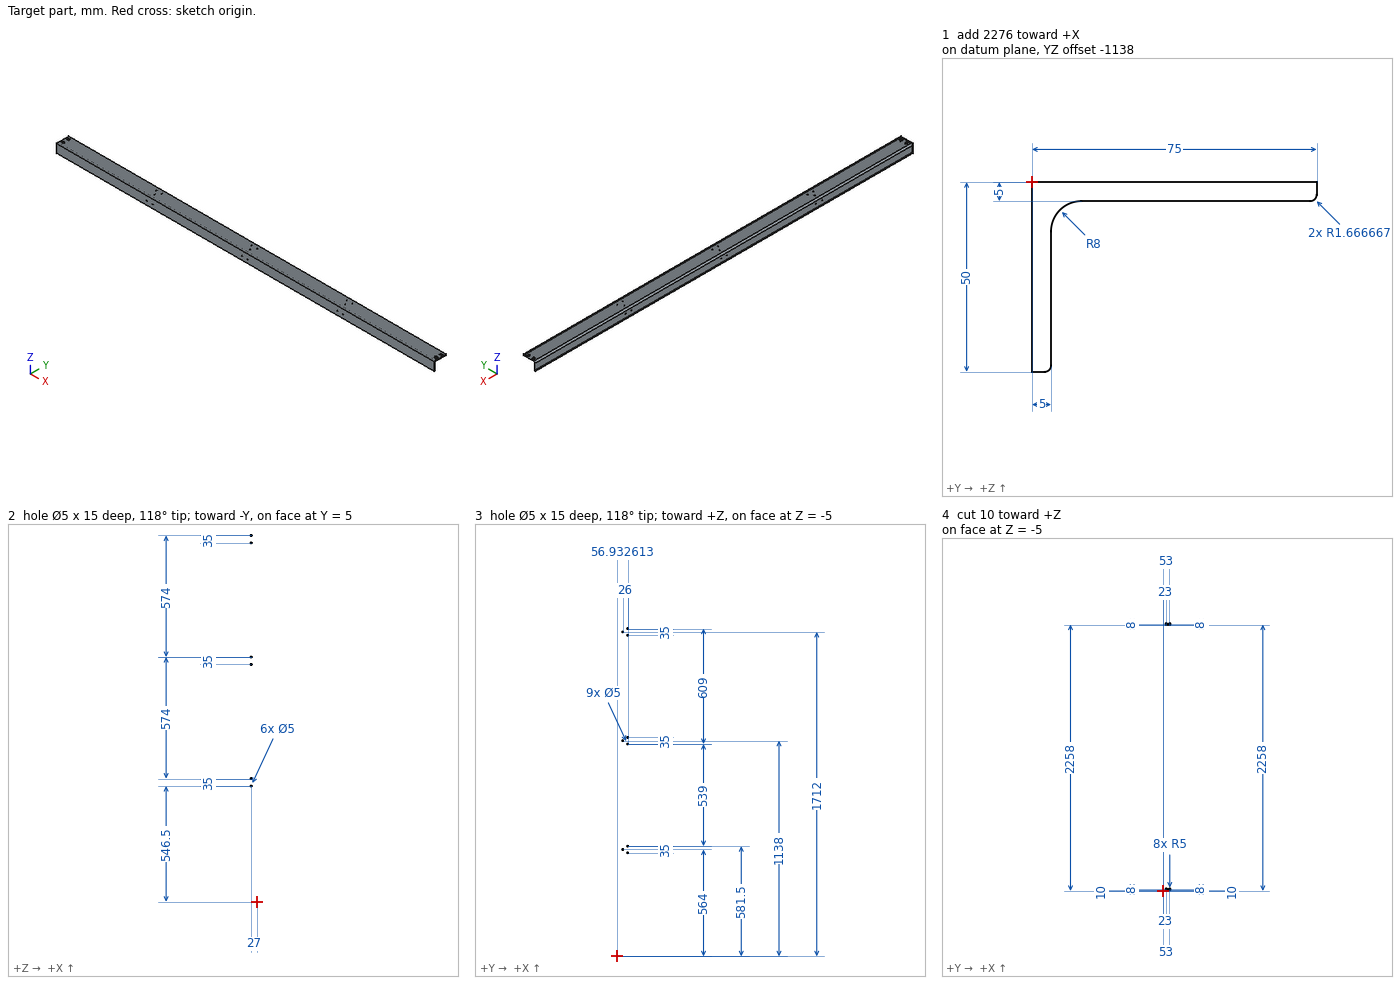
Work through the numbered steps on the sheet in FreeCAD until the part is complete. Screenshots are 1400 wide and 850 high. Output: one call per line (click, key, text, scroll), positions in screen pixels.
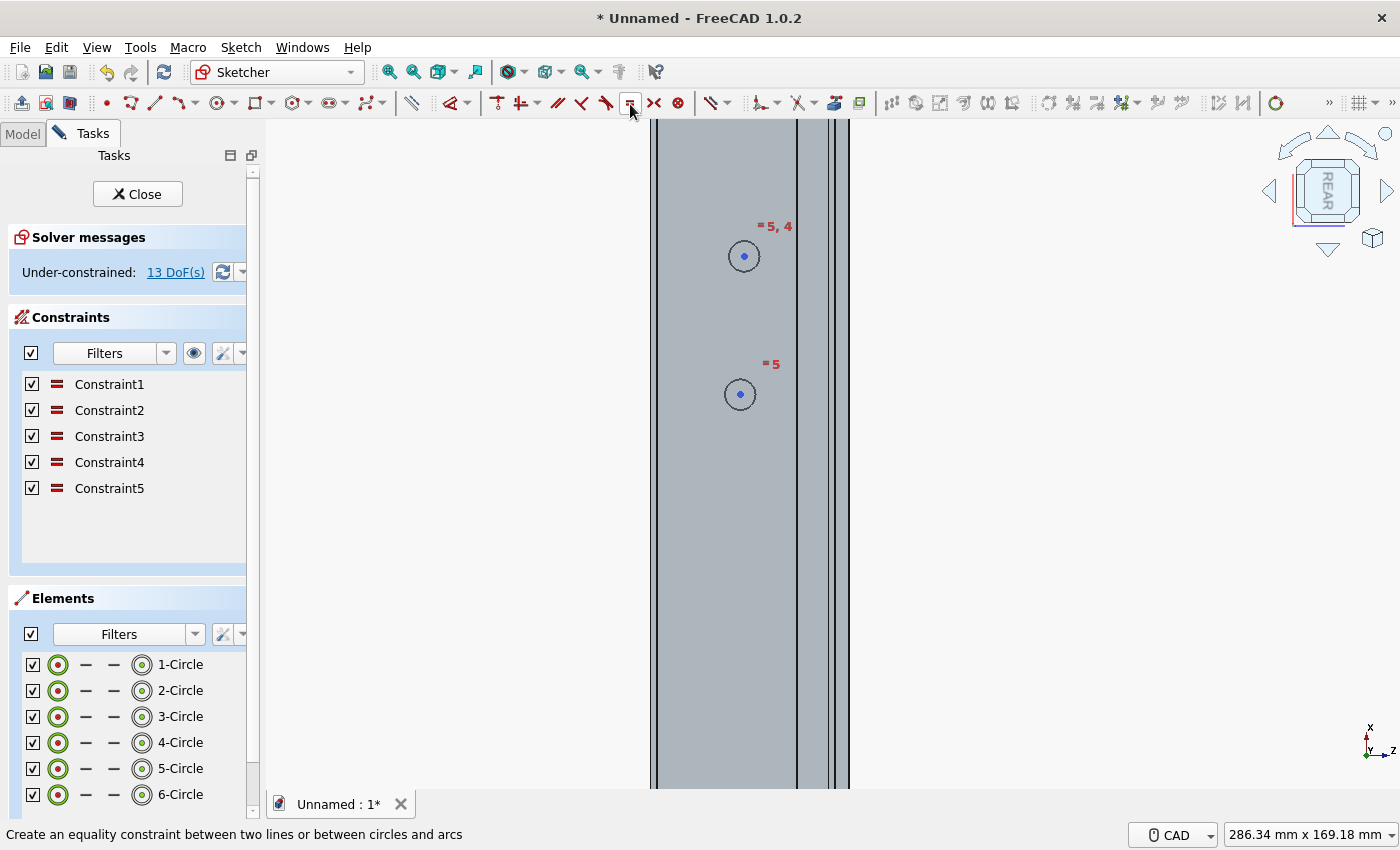
scroll(763, 246, down, 14)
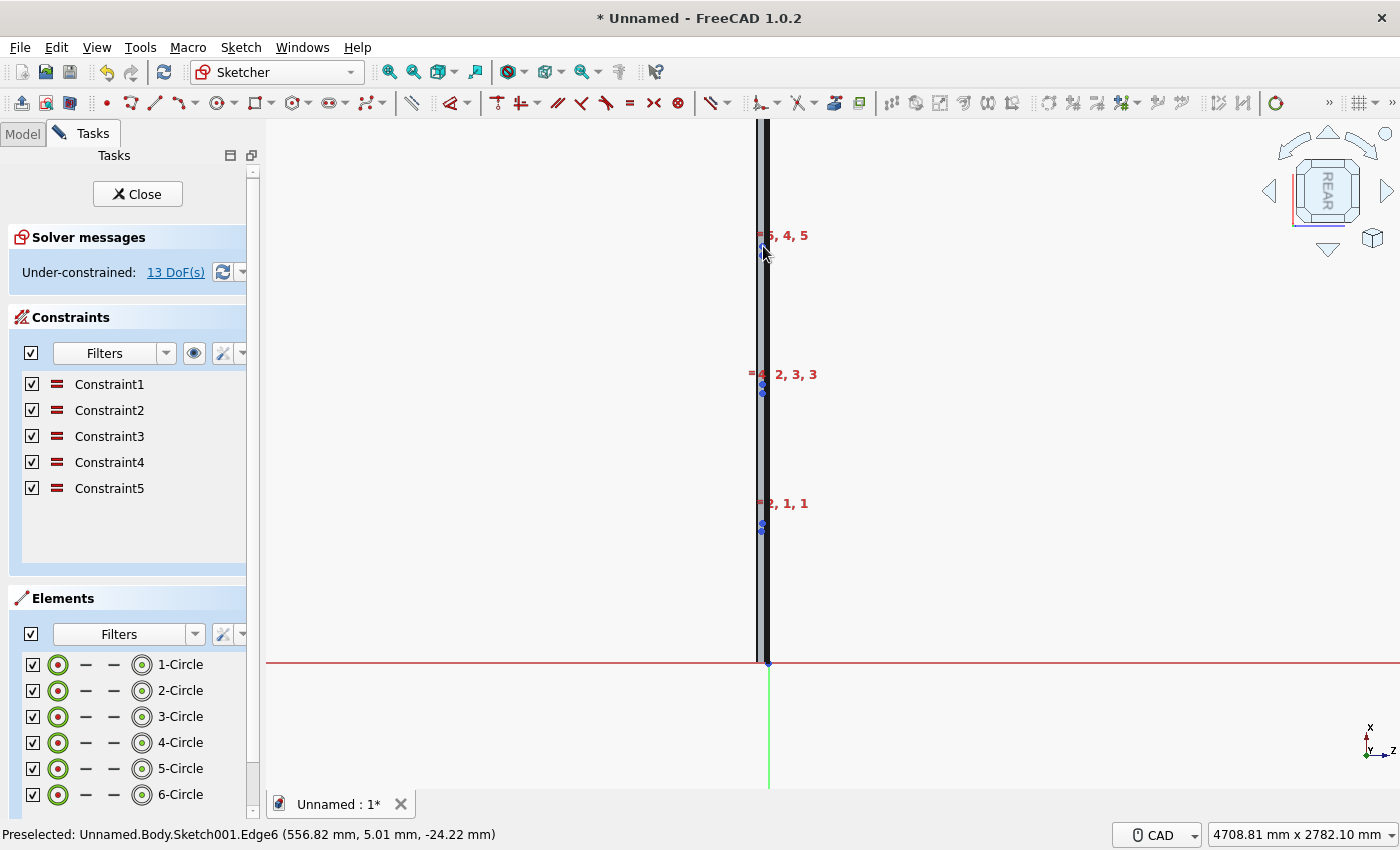
scroll(762, 532, up, 2)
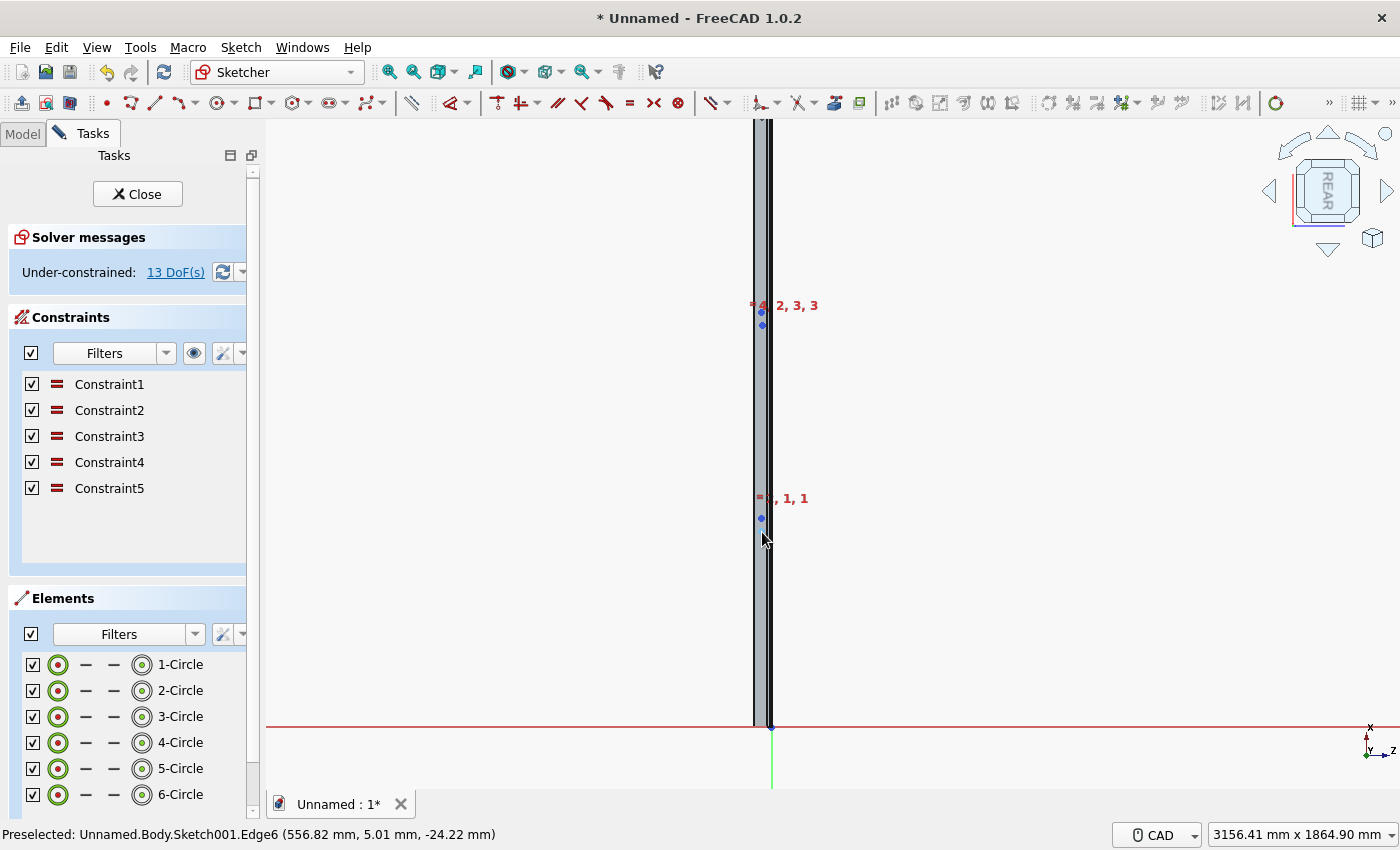
click(762, 531)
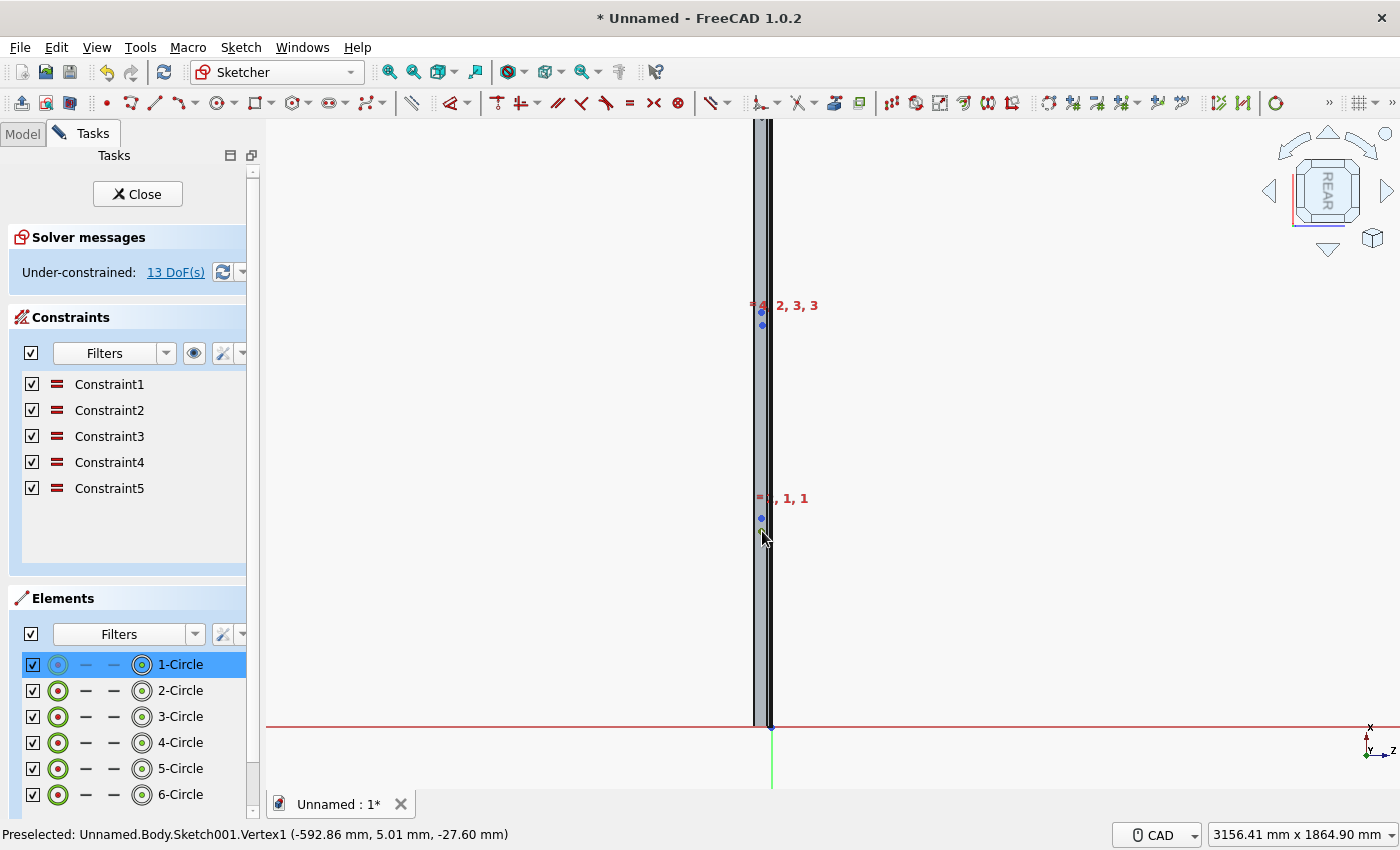
click(762, 519)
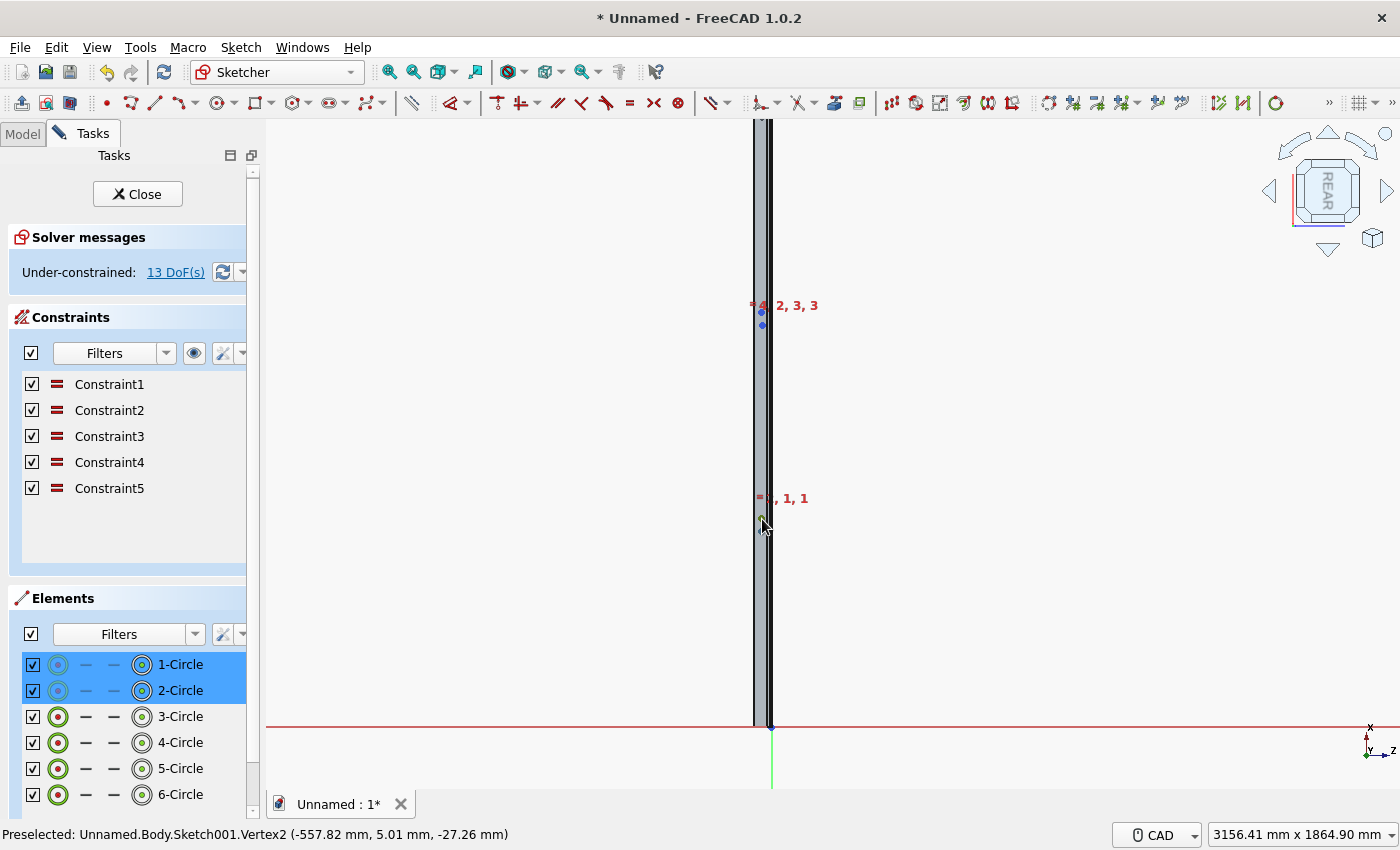
click(540, 104)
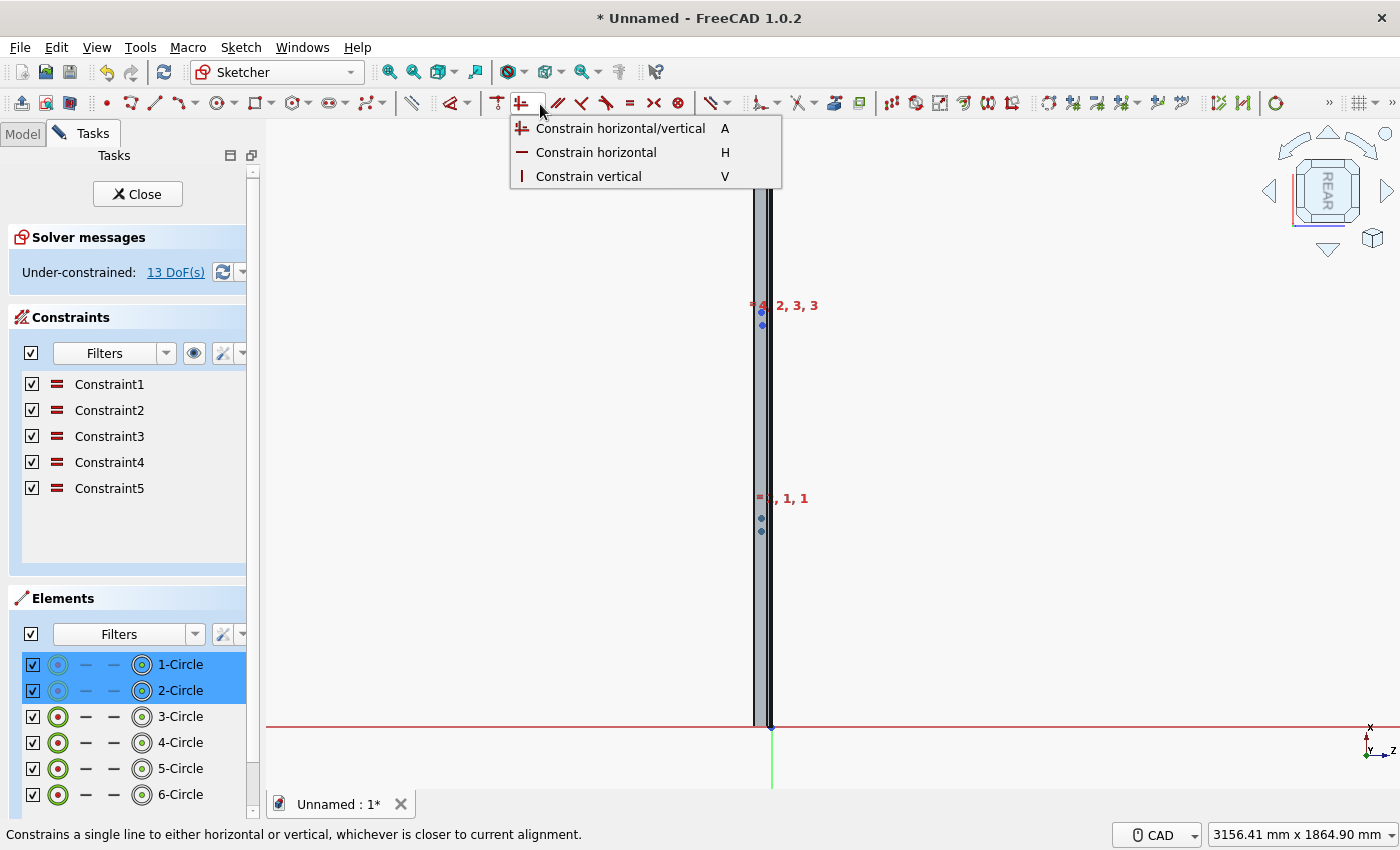
click(646, 176)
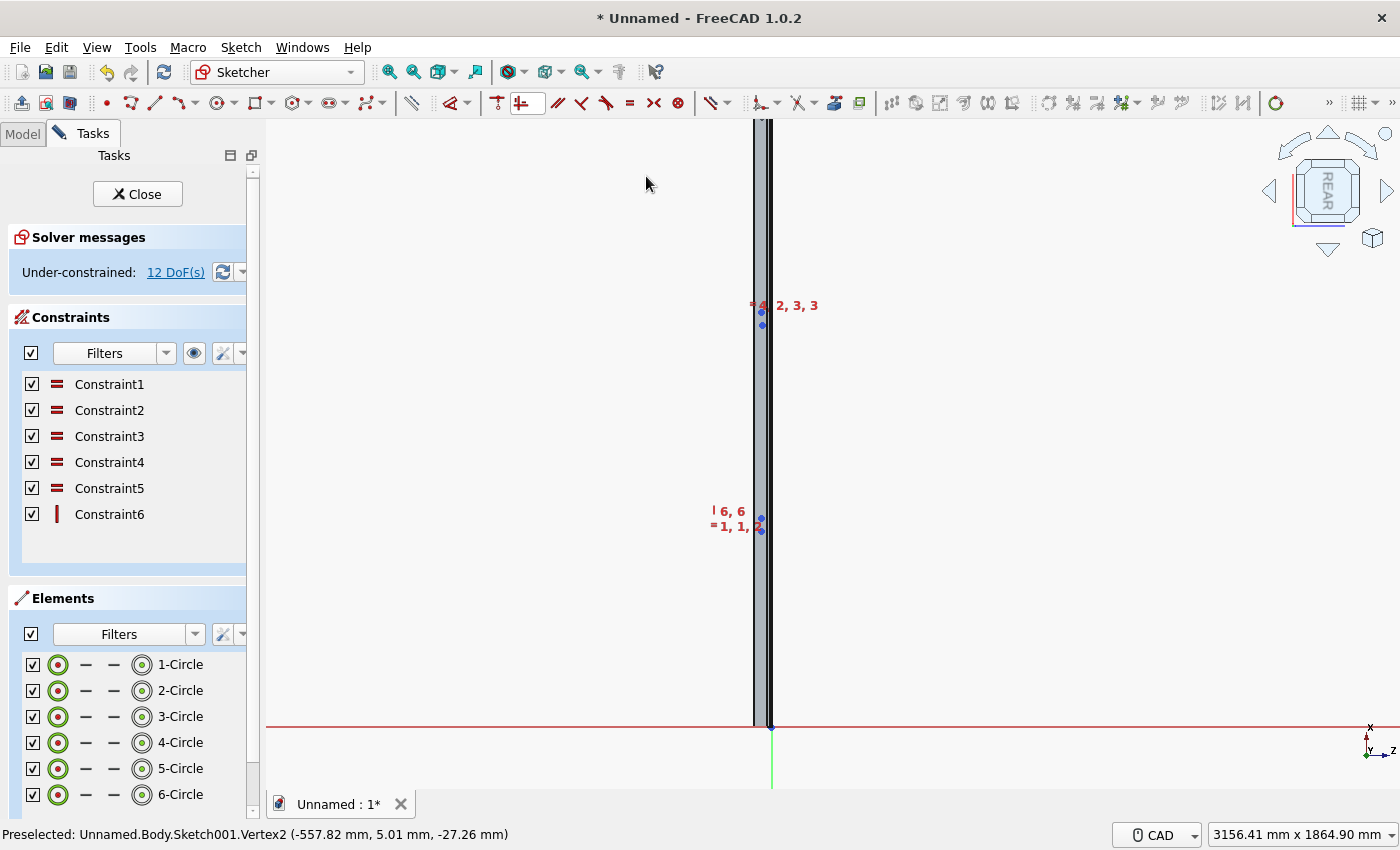
click(762, 519)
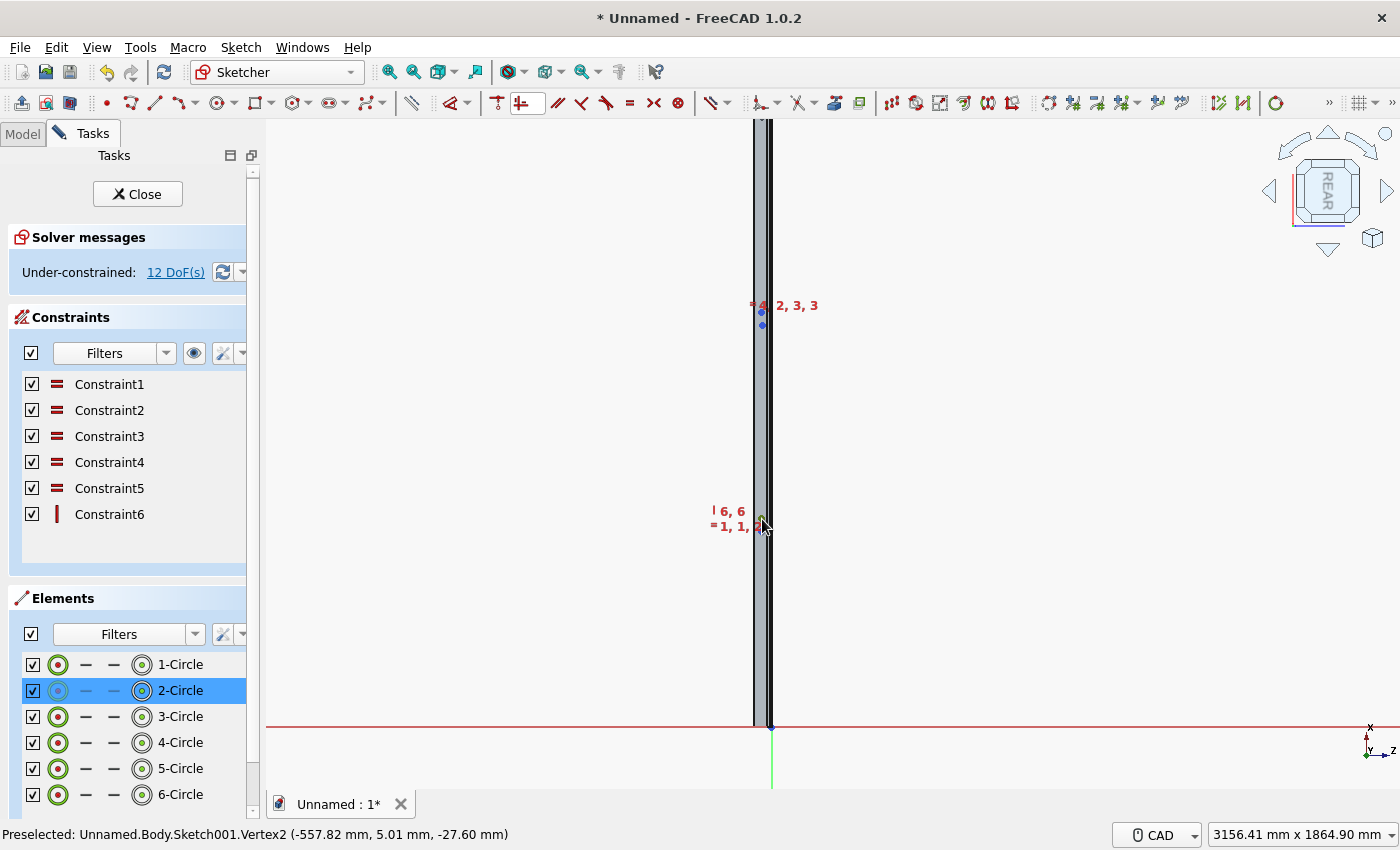
click(762, 312)